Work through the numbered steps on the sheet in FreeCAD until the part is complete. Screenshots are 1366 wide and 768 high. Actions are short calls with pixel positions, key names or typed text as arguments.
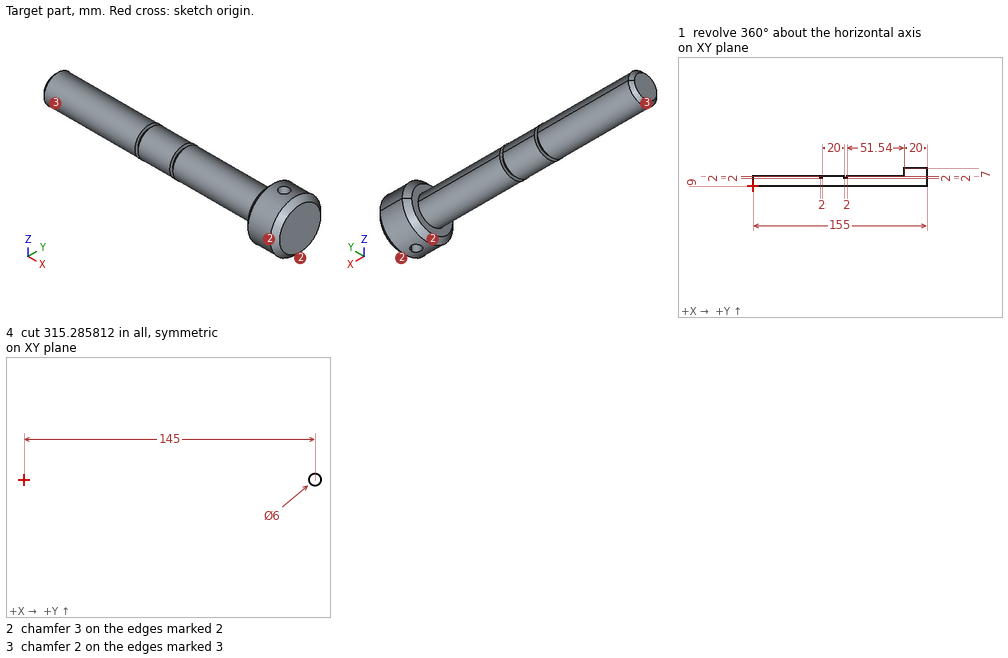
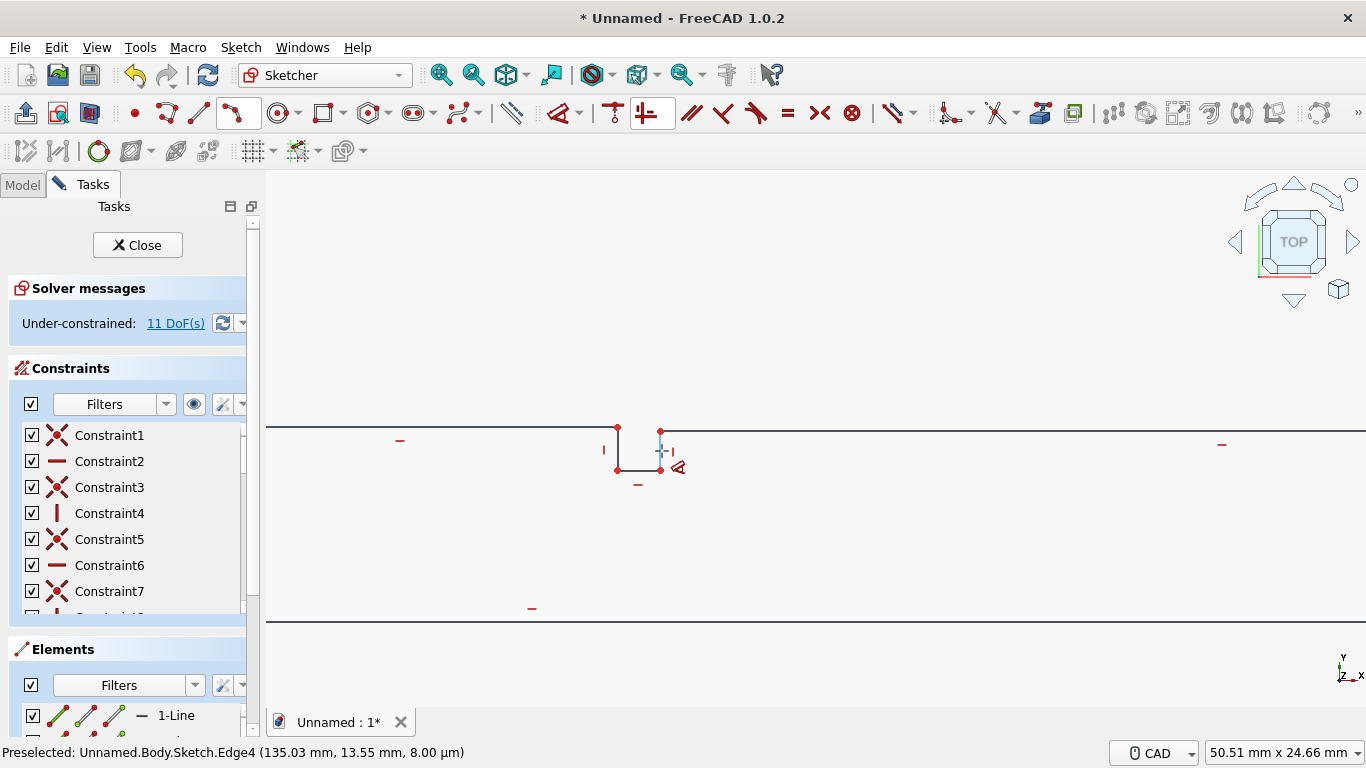
click(660, 451)
click(694, 451)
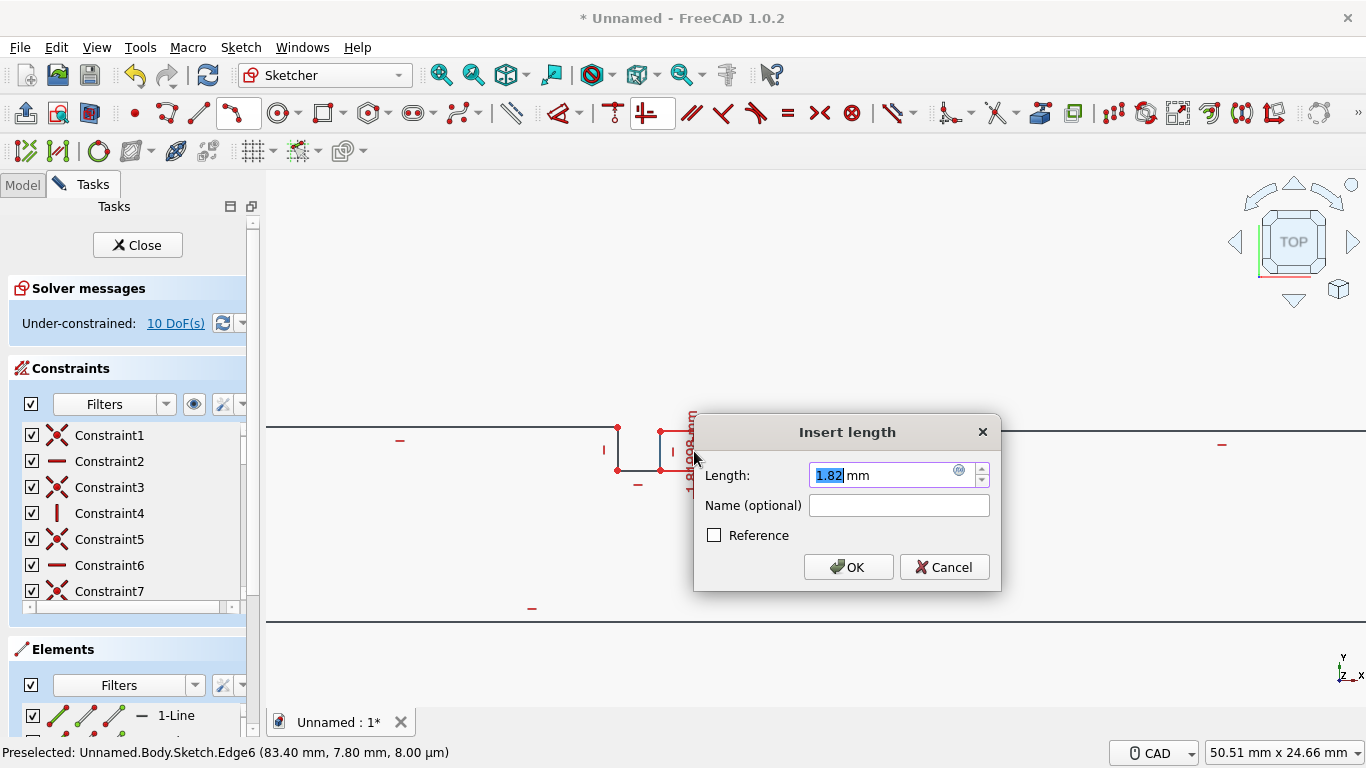
text(2)
key(Return)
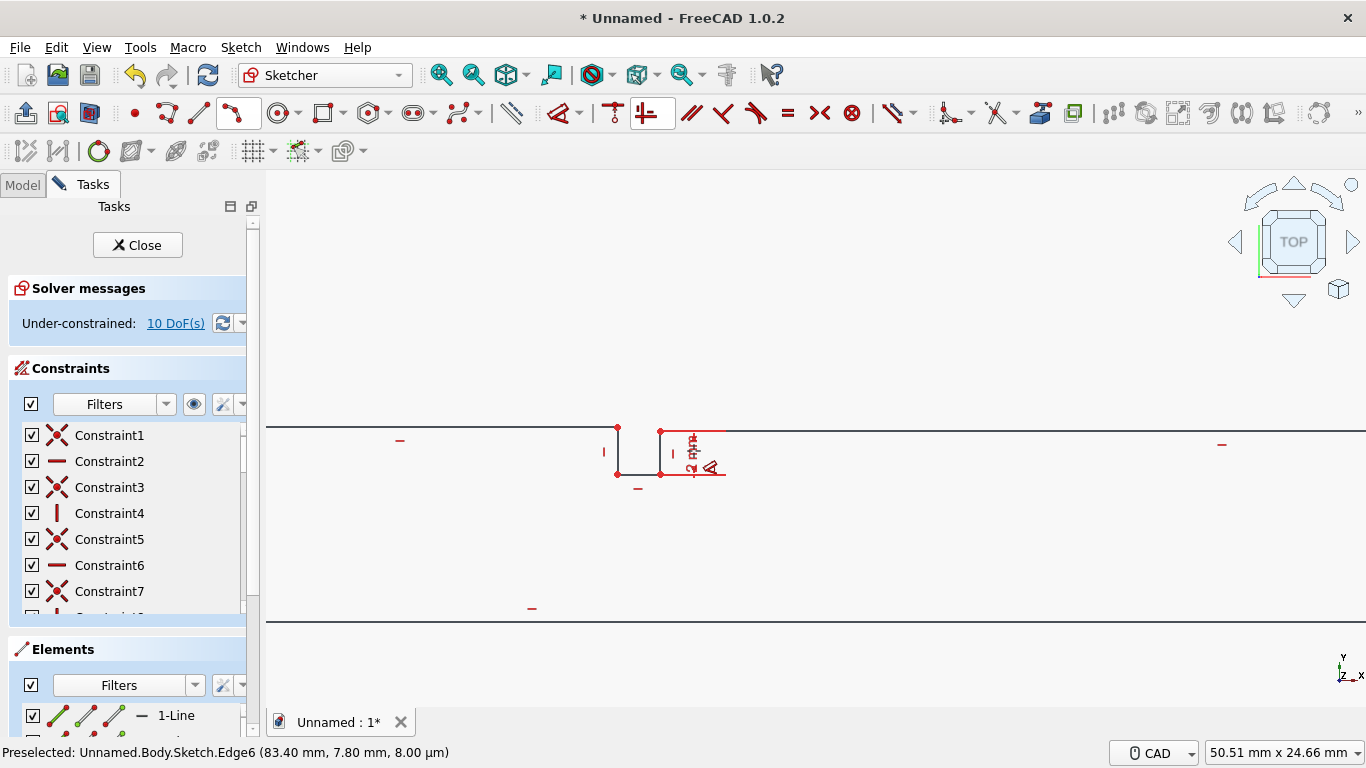
click(647, 475)
click(639, 509)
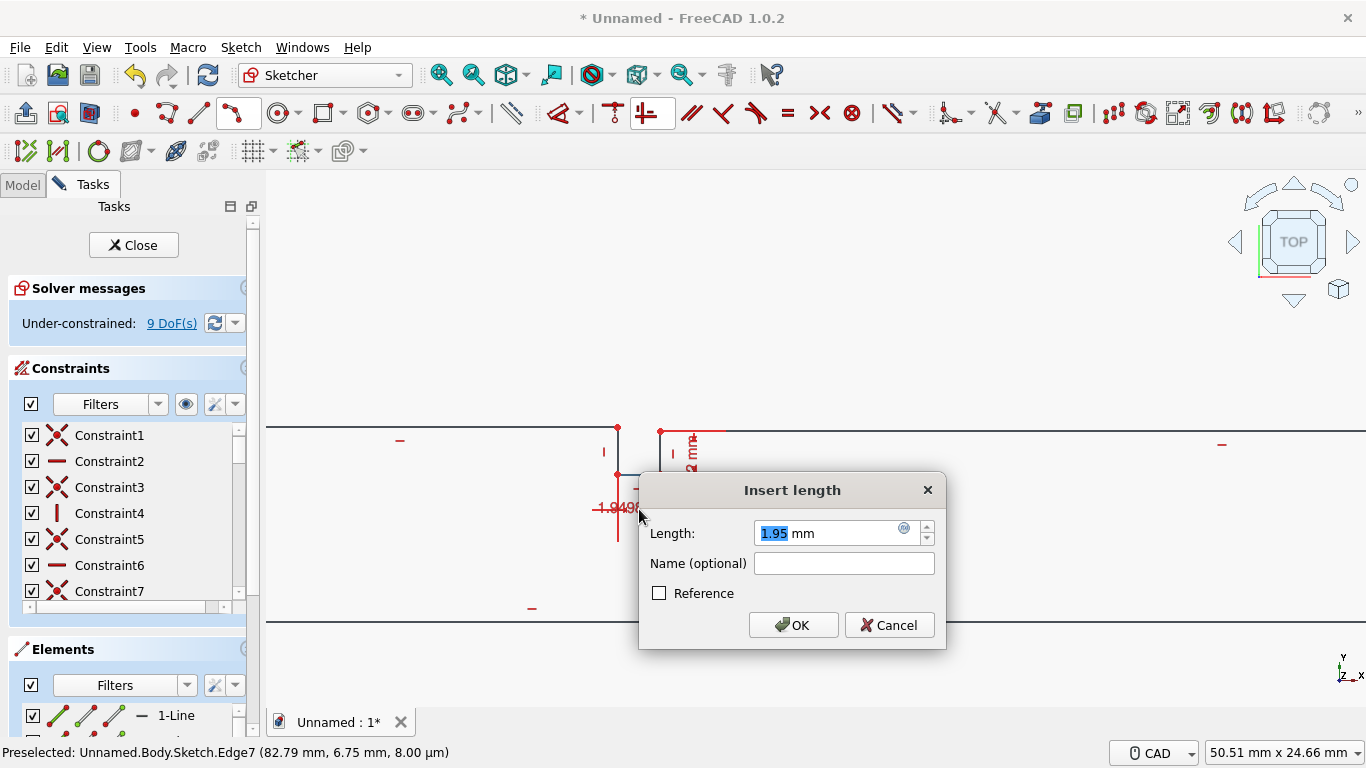
text(2)
key(Return)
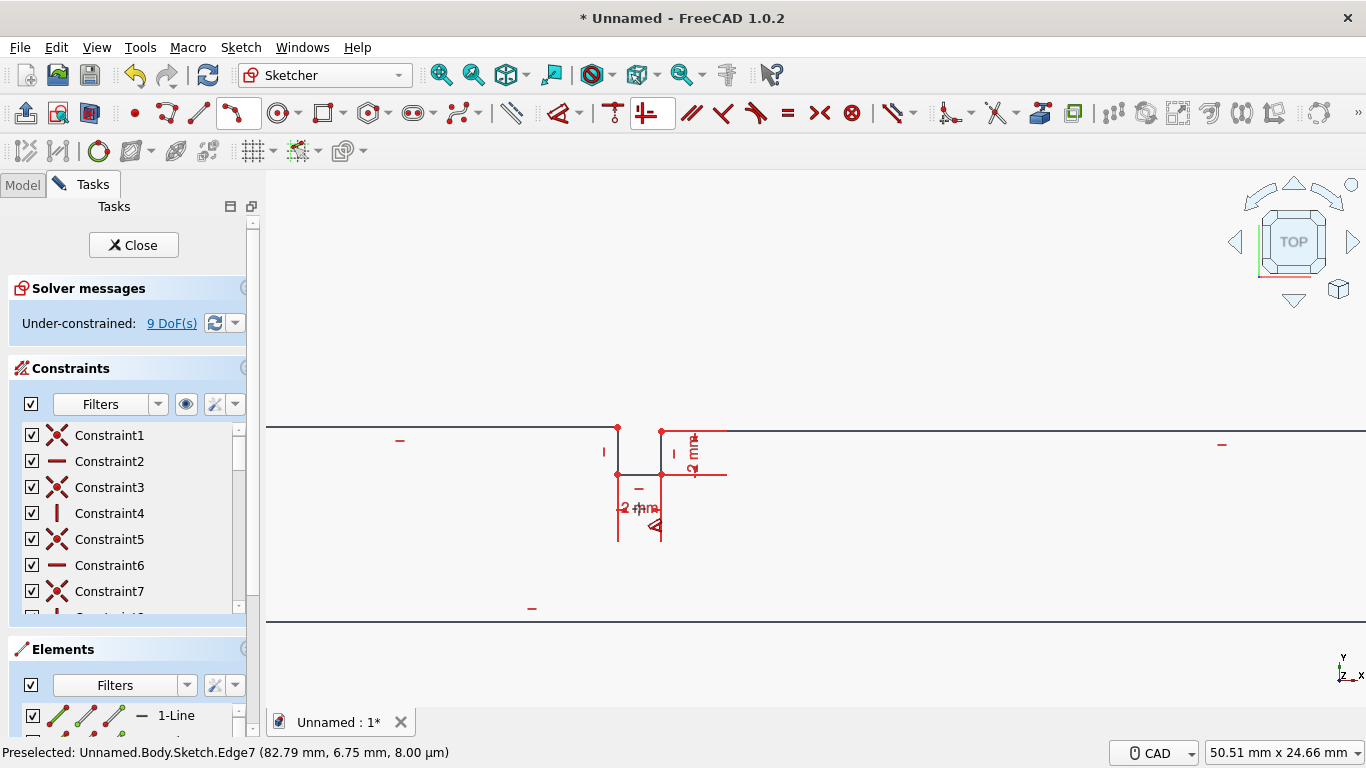
click(618, 461)
click(584, 451)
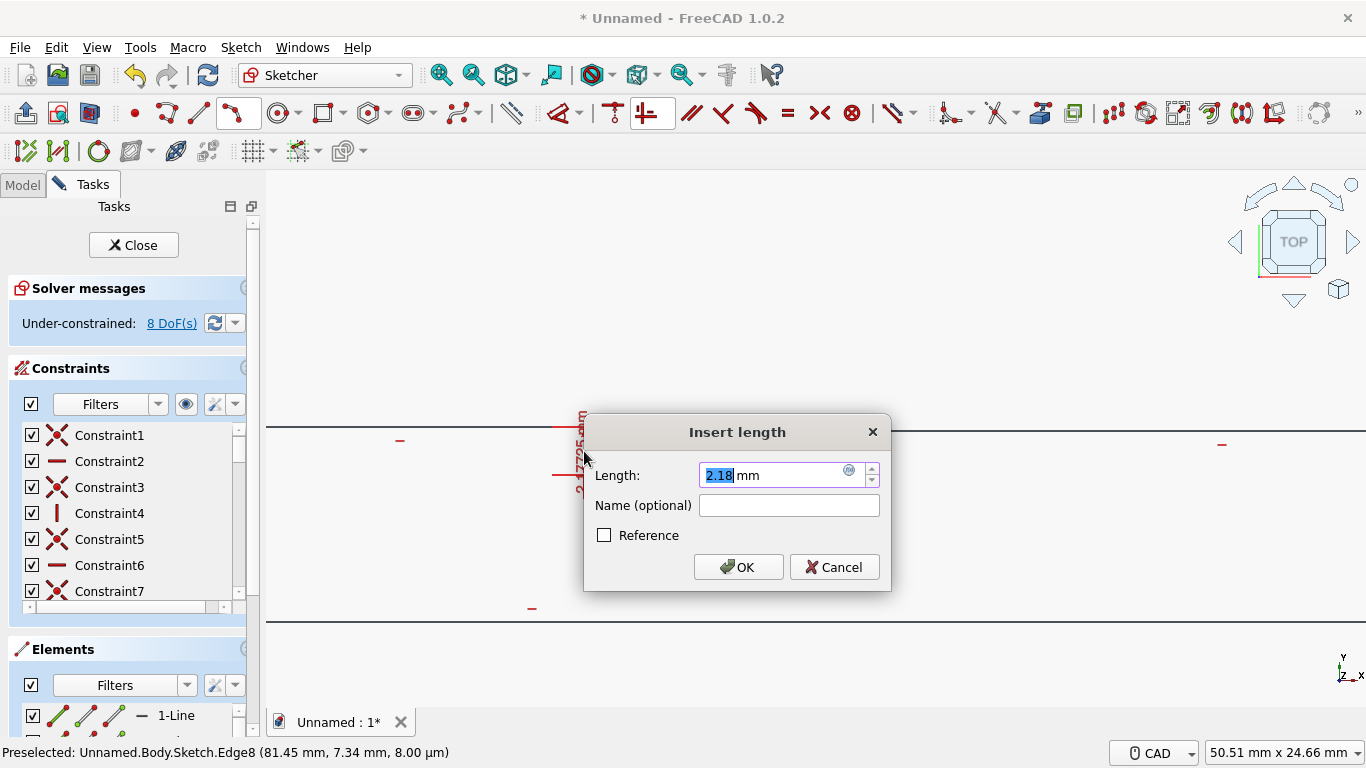
text(2)
key(Return)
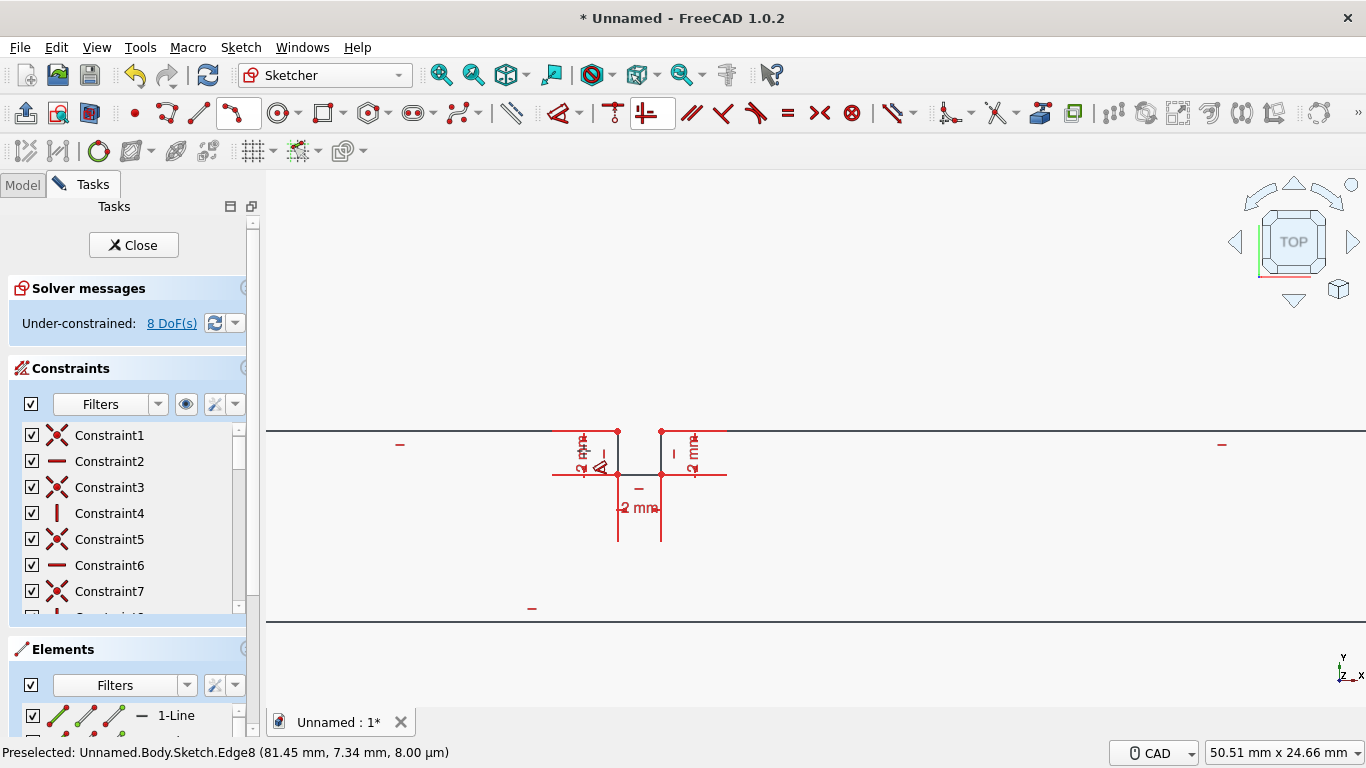
scroll(802, 436, down, 8)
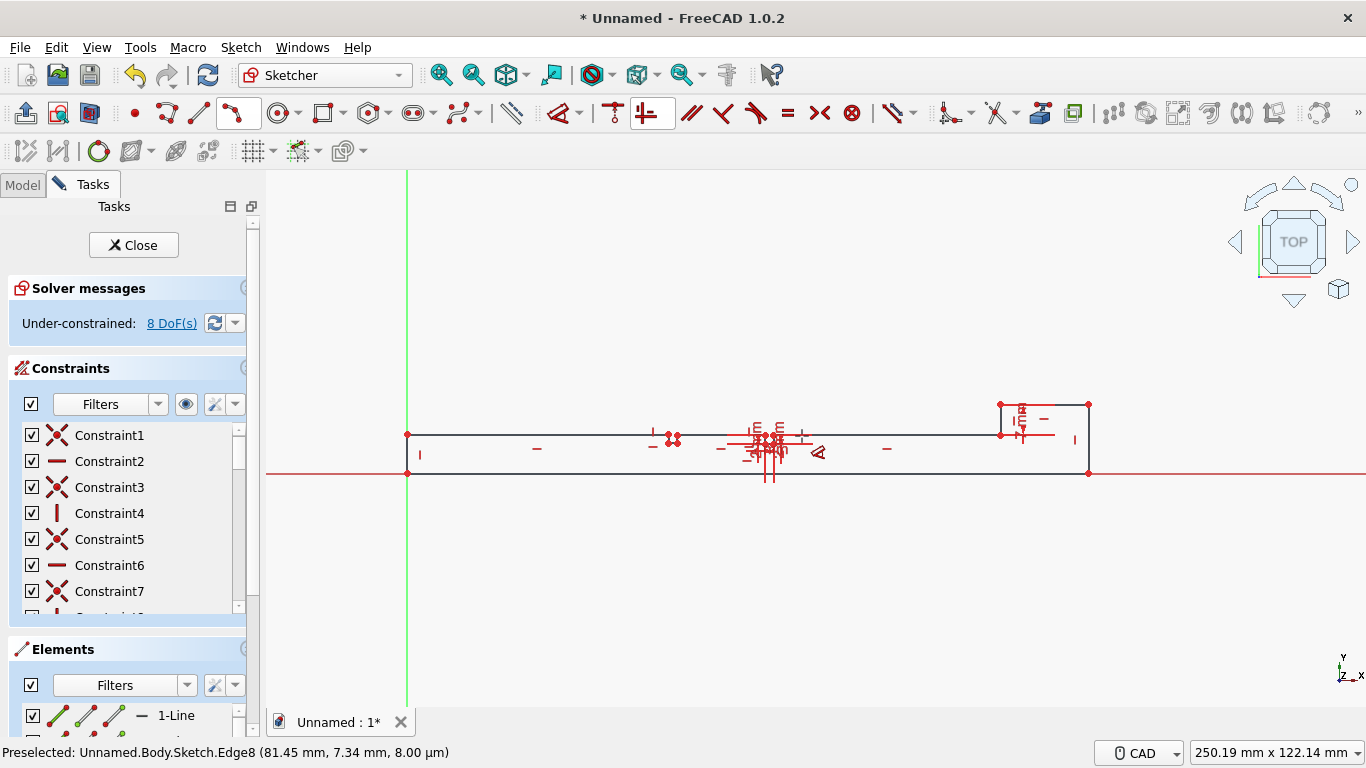
scroll(677, 438, up, 9)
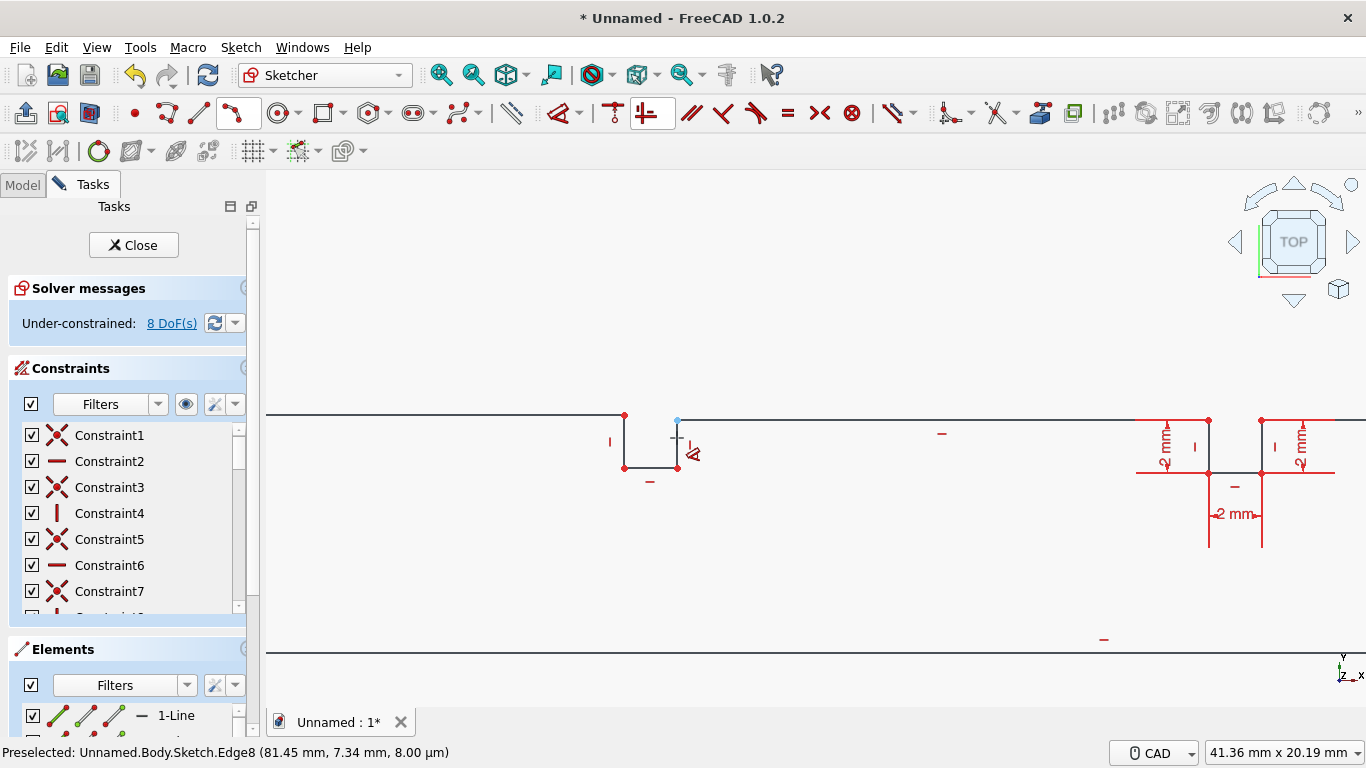
click(677, 435)
click(643, 444)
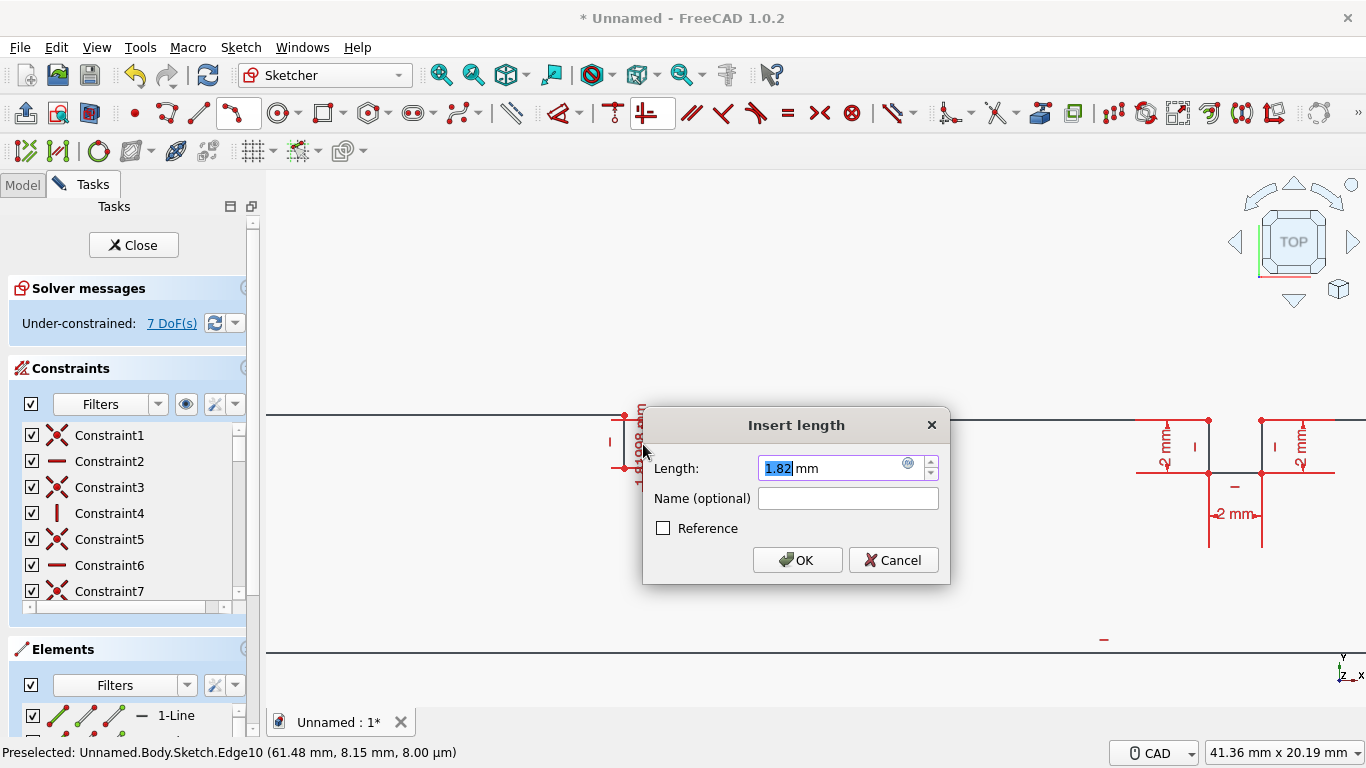
text(2)
key(Return)